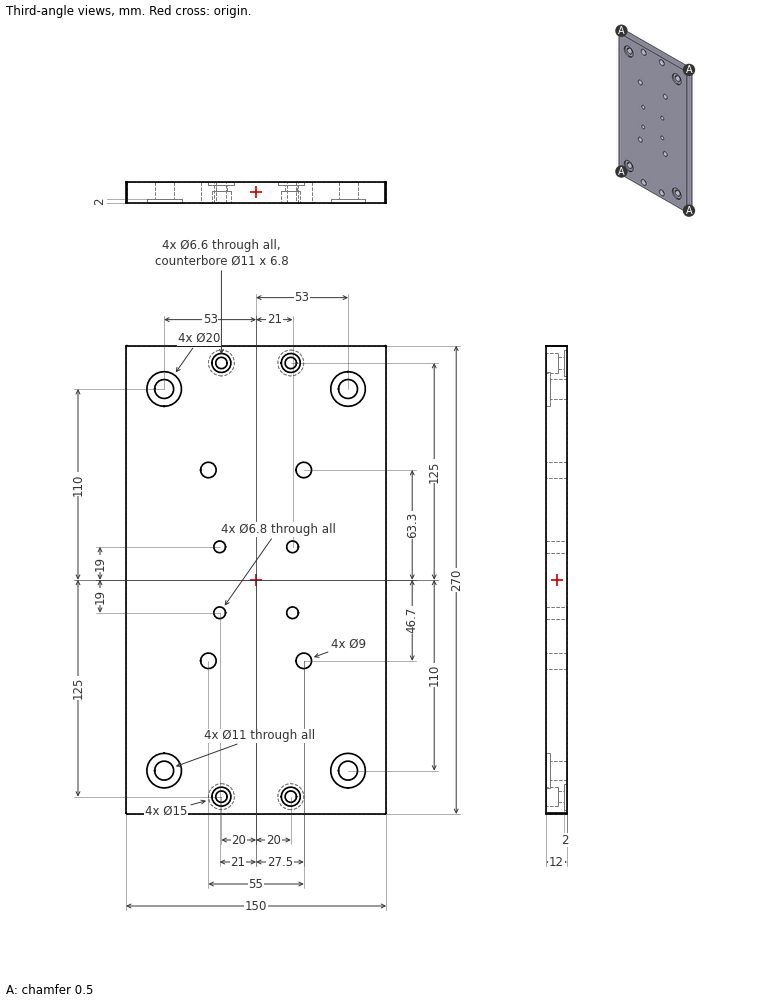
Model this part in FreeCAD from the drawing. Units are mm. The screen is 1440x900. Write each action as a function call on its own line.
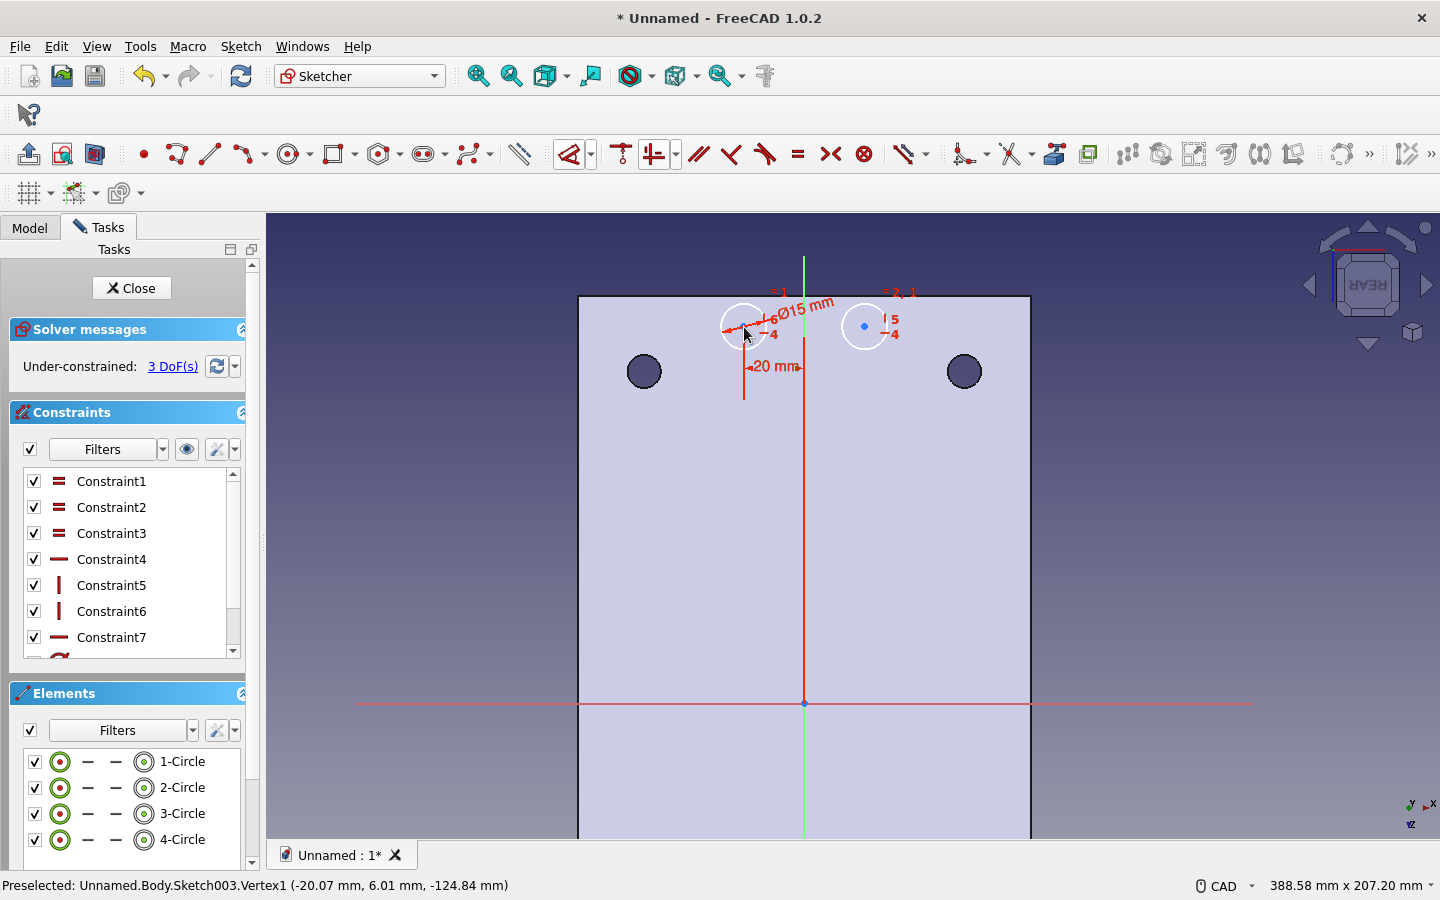
click(865, 327)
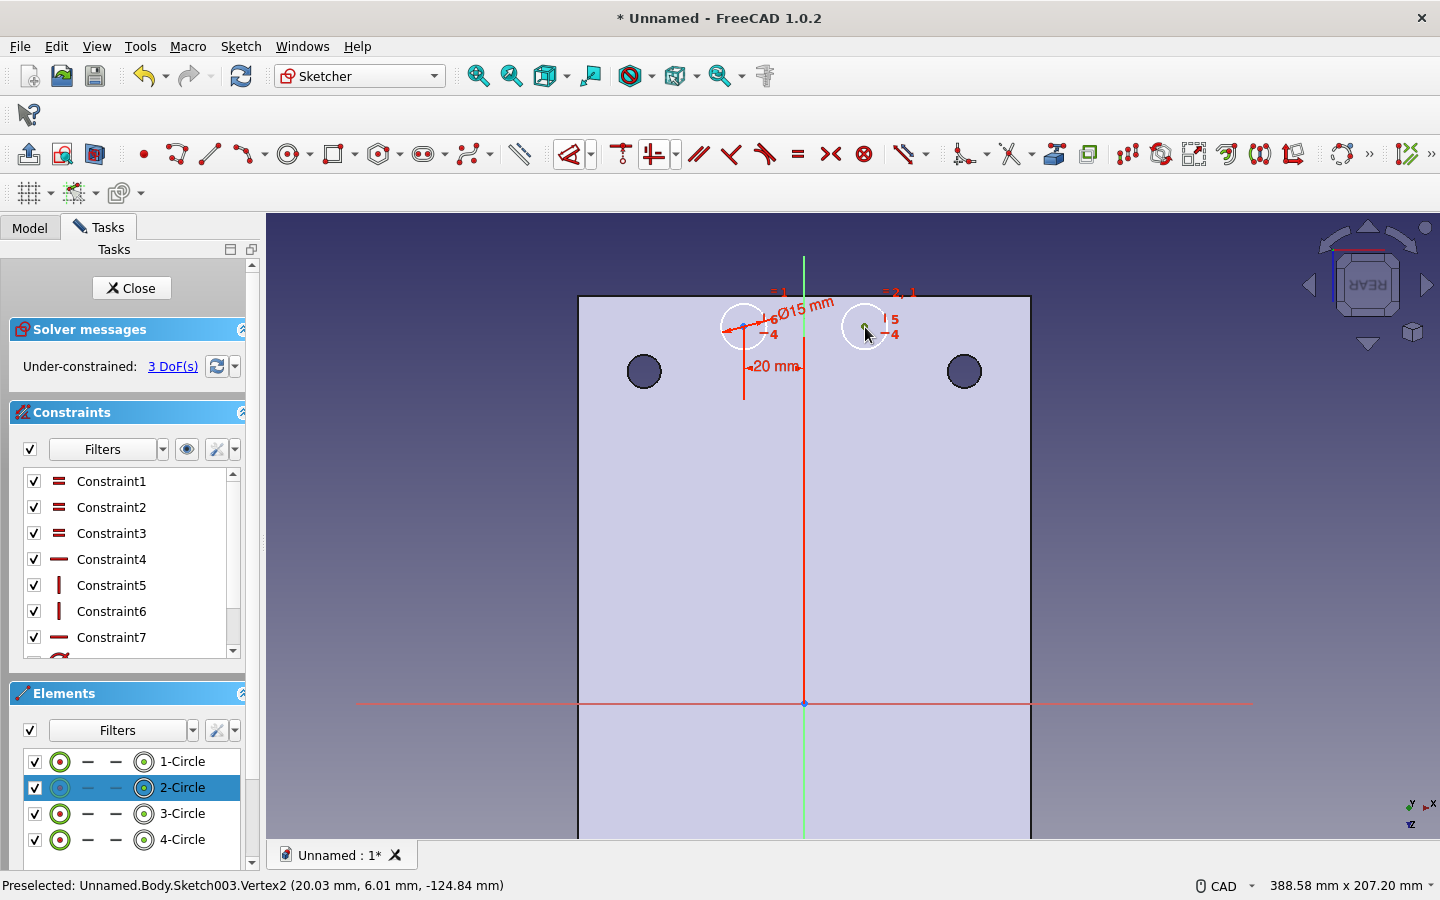
key(l)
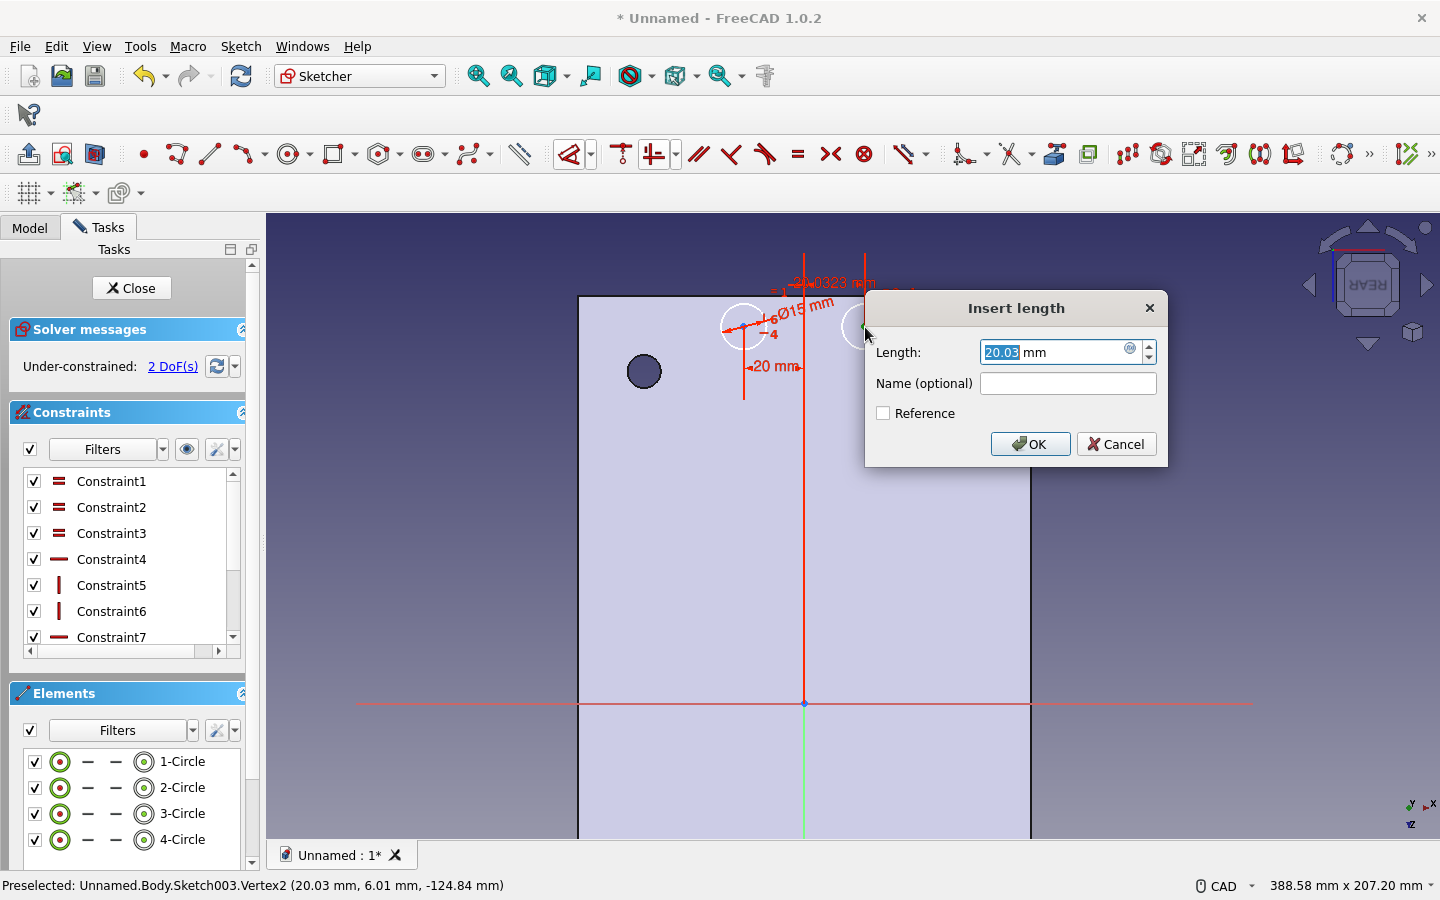
text(20)
key(Return)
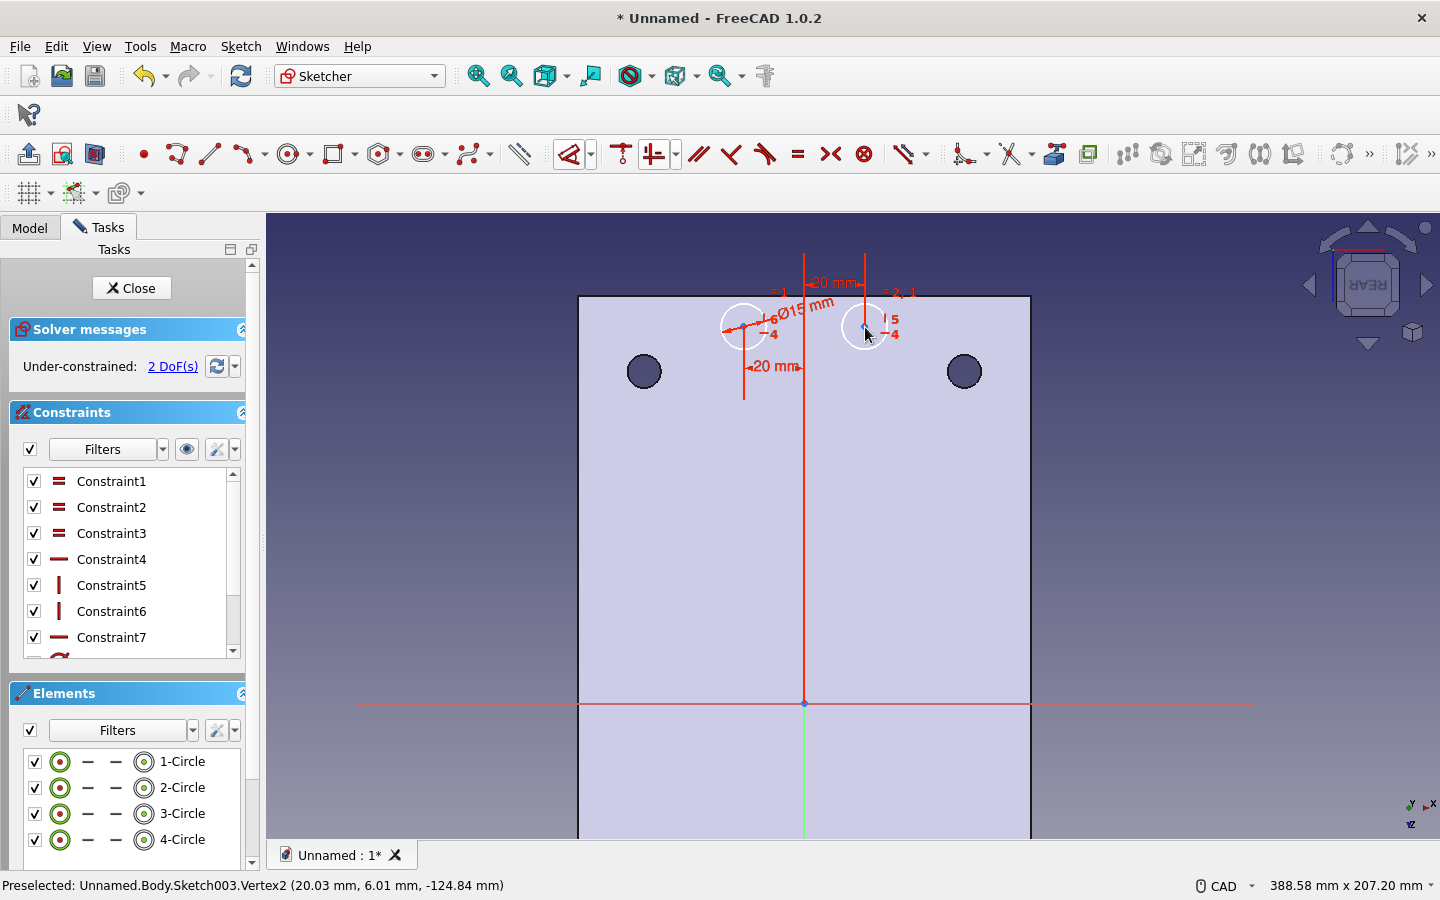
click(744, 327)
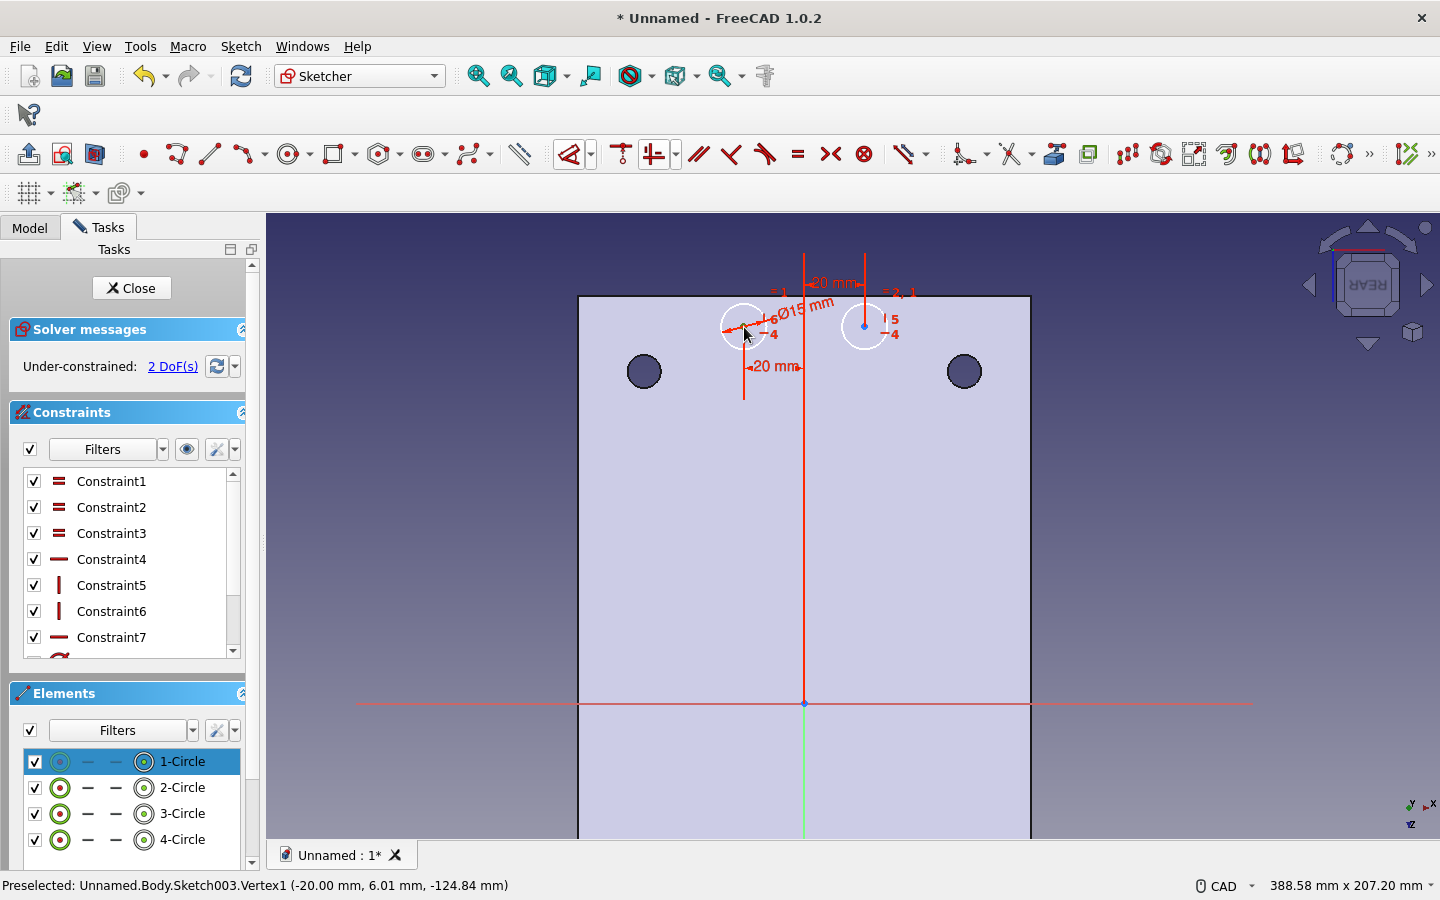
key(i)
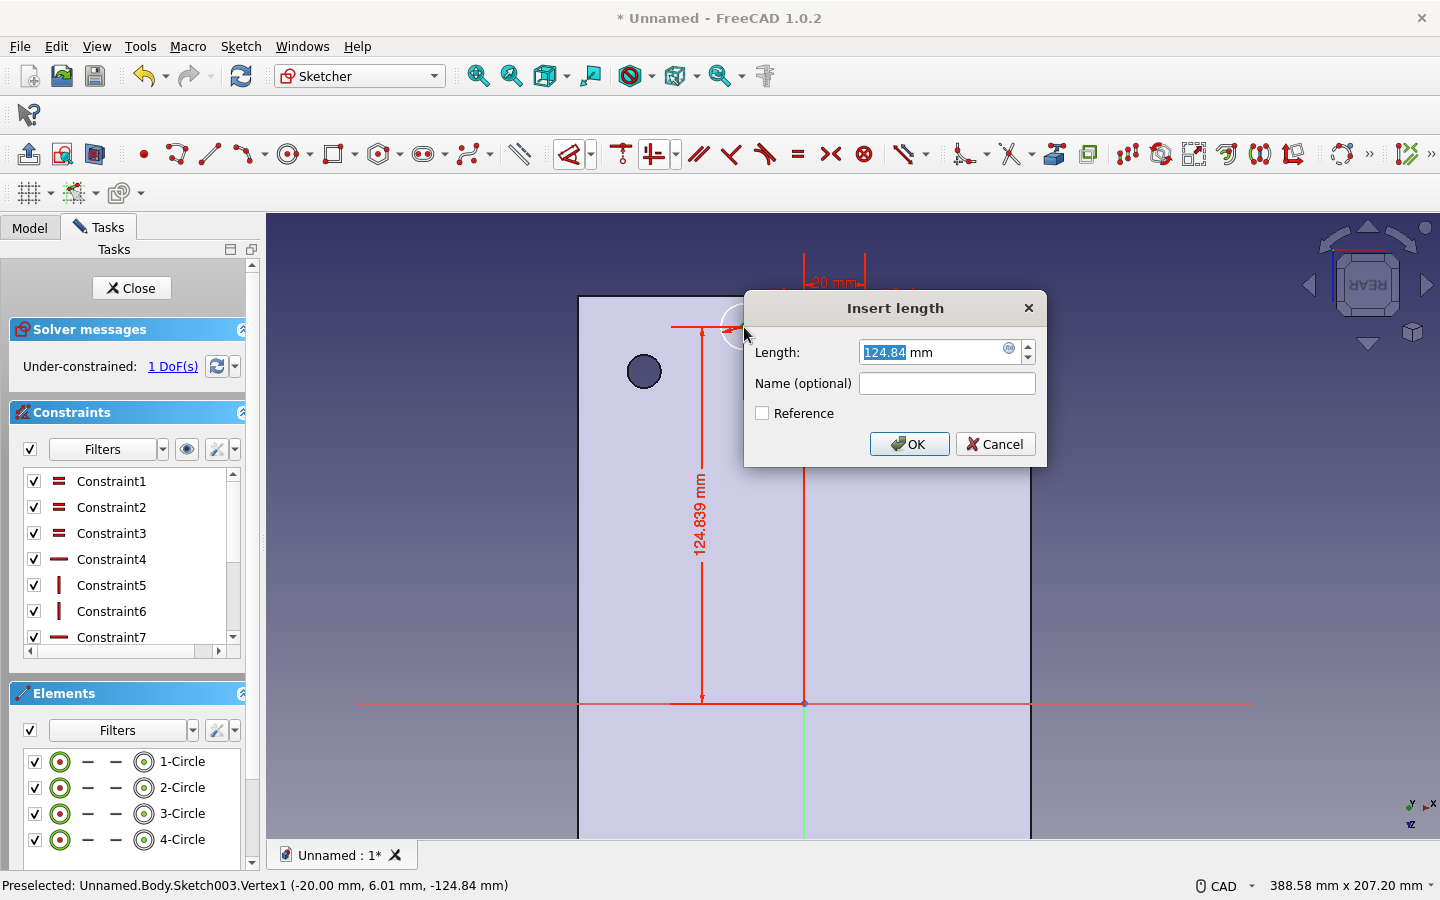
text(125)
key(Return)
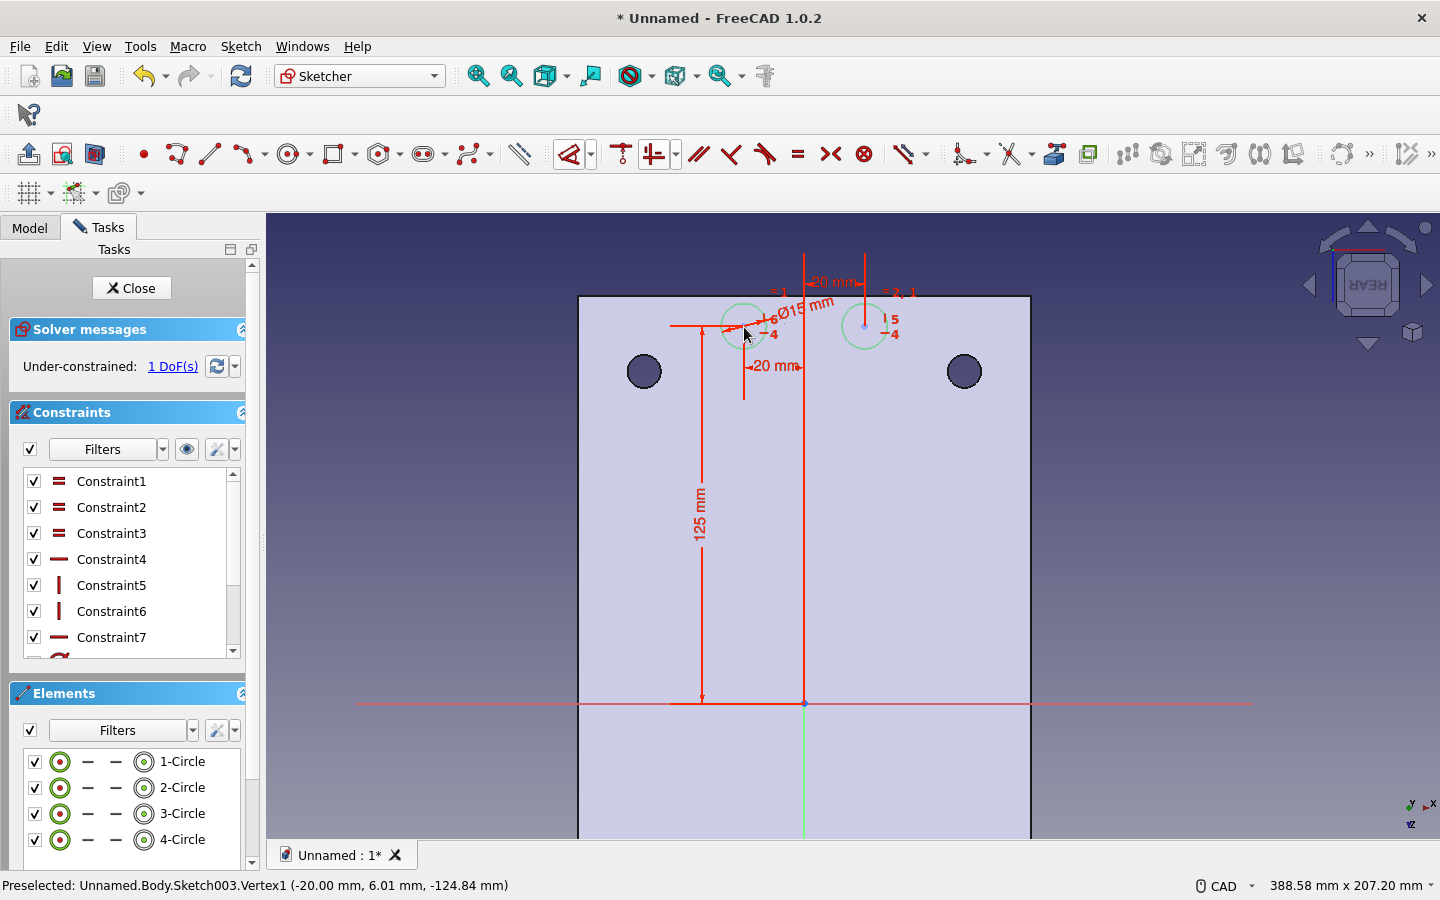
scroll(760, 310, down, 3)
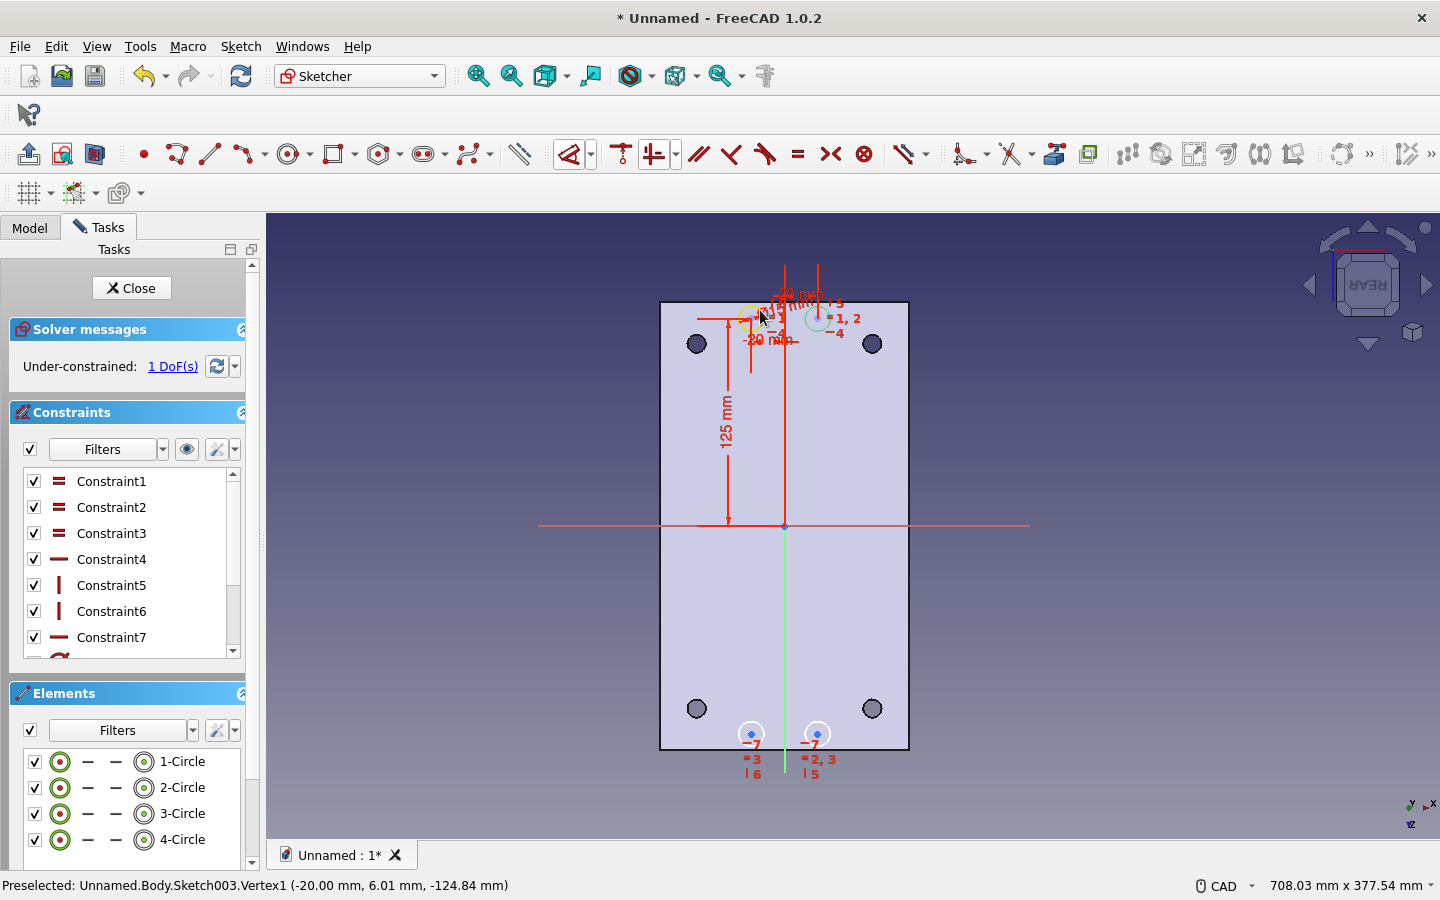
click(818, 734)